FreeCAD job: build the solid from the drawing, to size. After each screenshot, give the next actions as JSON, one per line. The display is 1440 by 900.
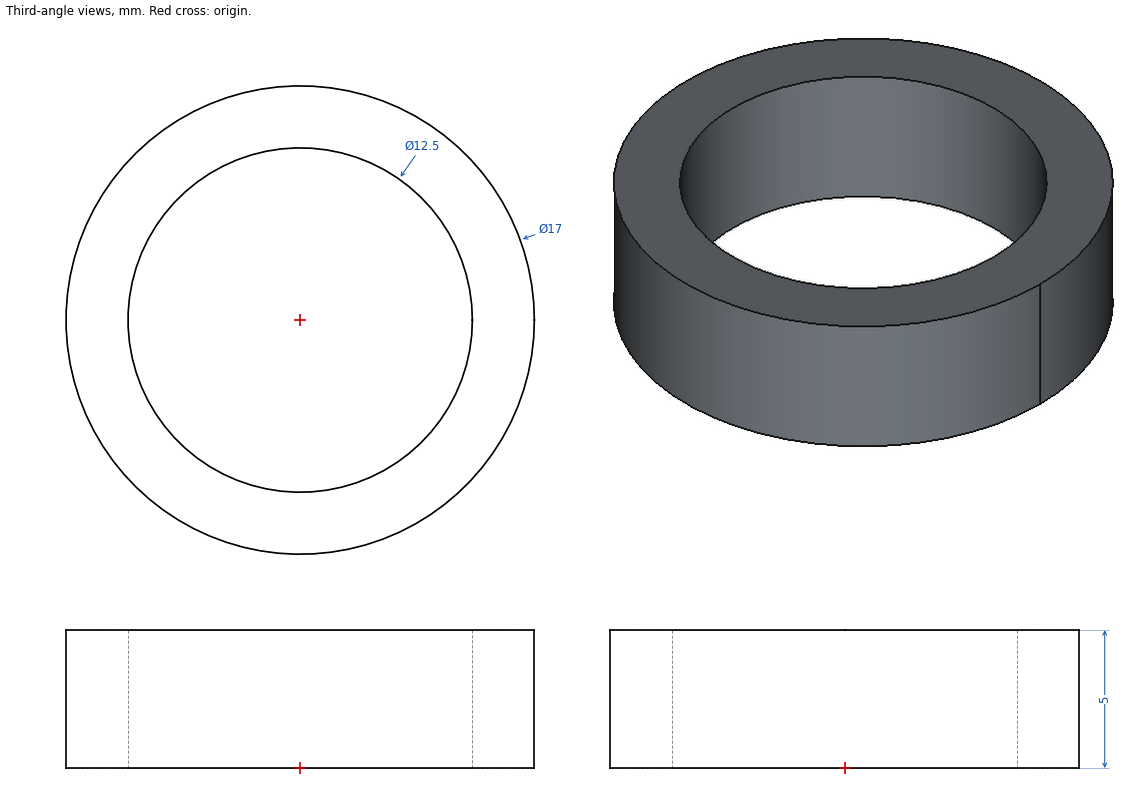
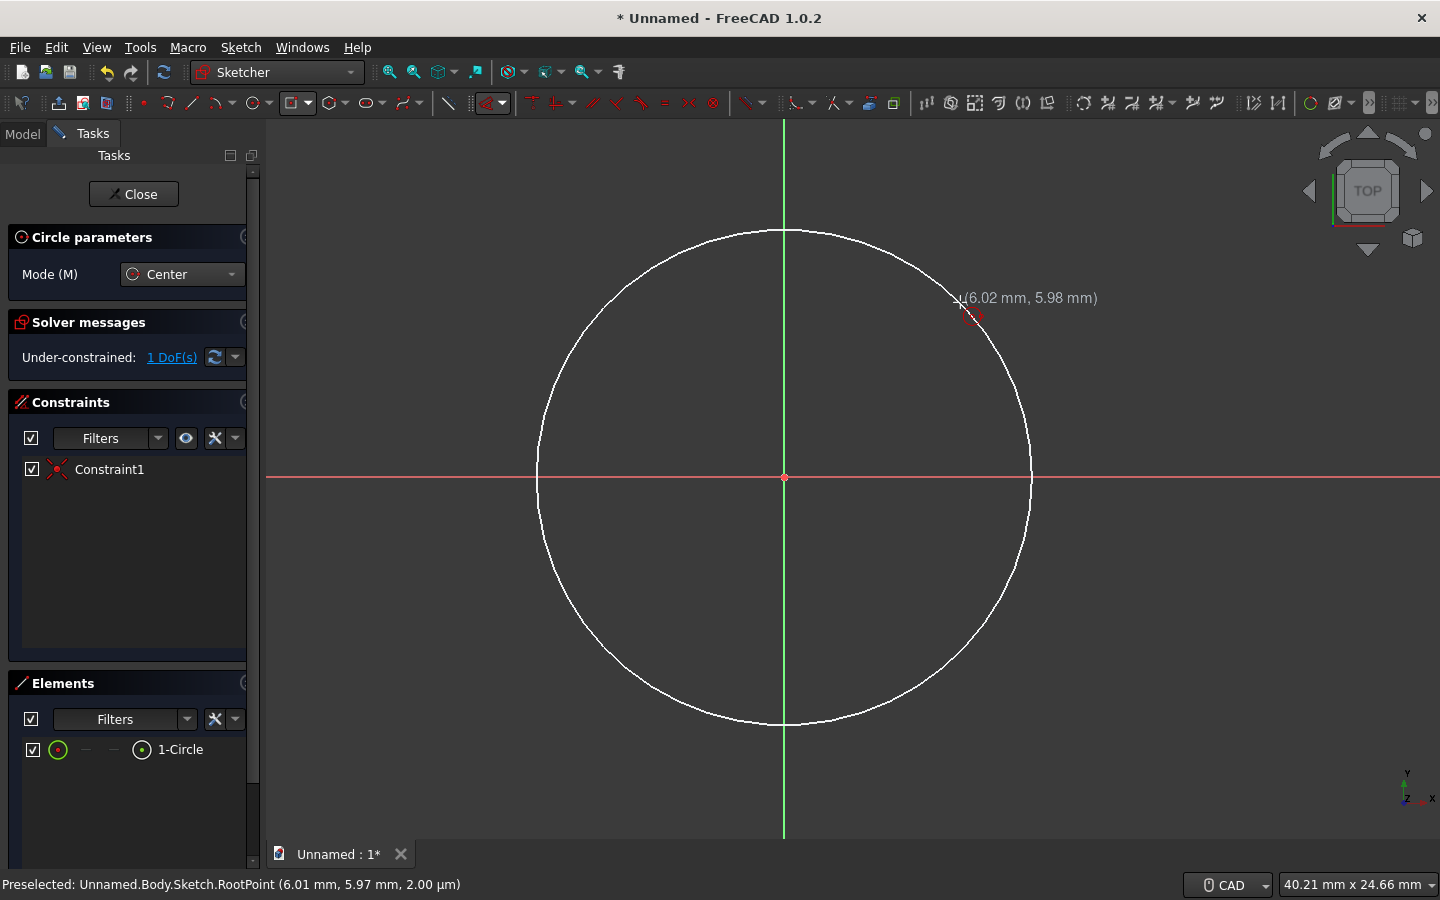
{"action": "left_click", "coordinate": [784, 477]}
{"action": "left_click", "coordinate": [913, 348]}
{"action": "key", "text": "Escape"}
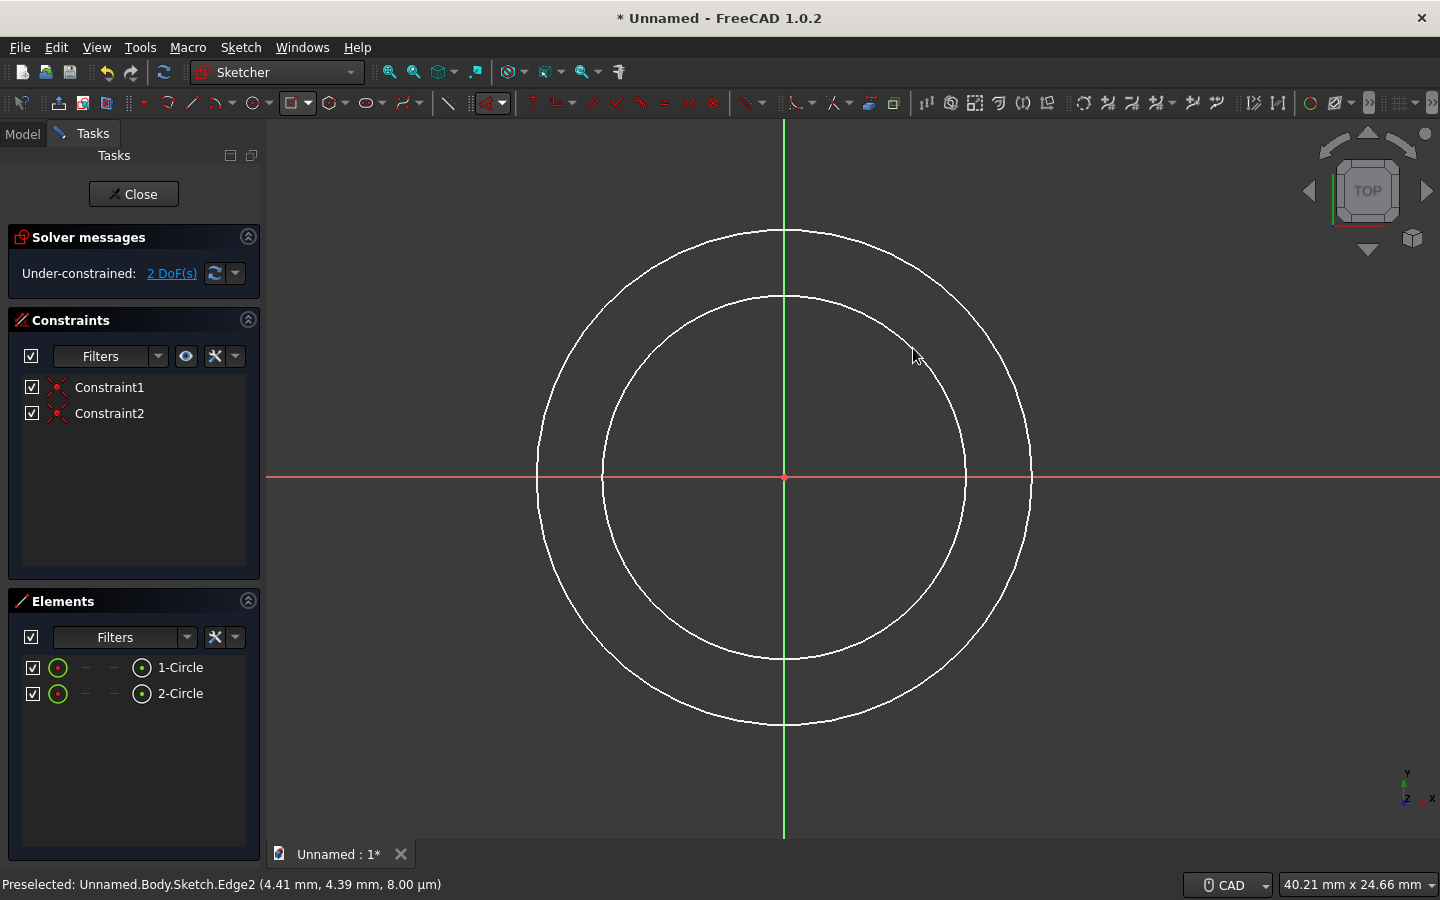
{"action": "key", "text": "d"}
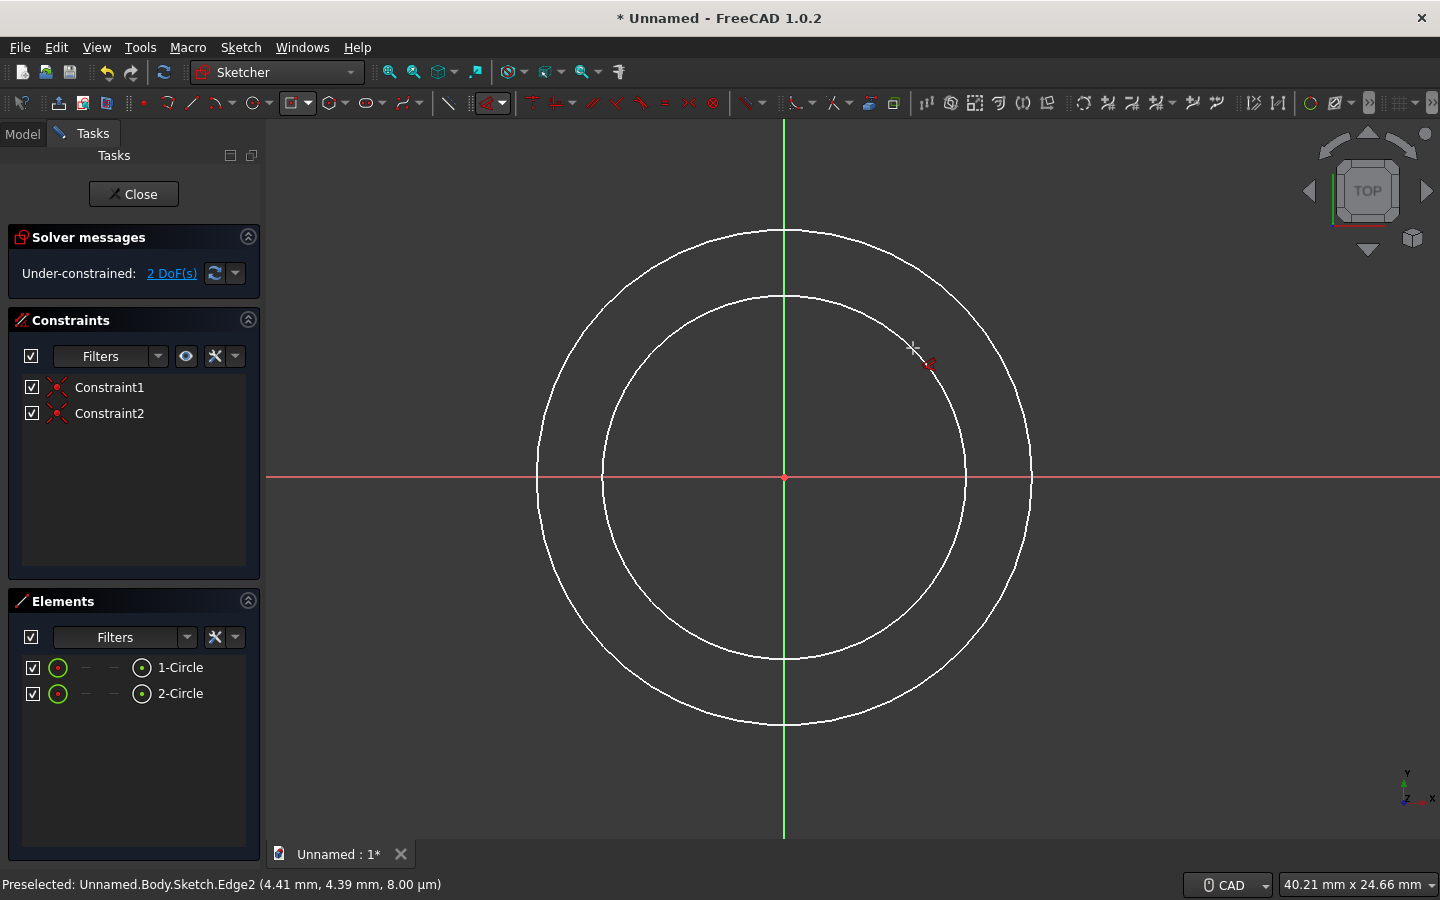
{"action": "left_click", "coordinate": [959, 302]}
{"action": "left_click", "coordinate": [982, 279]}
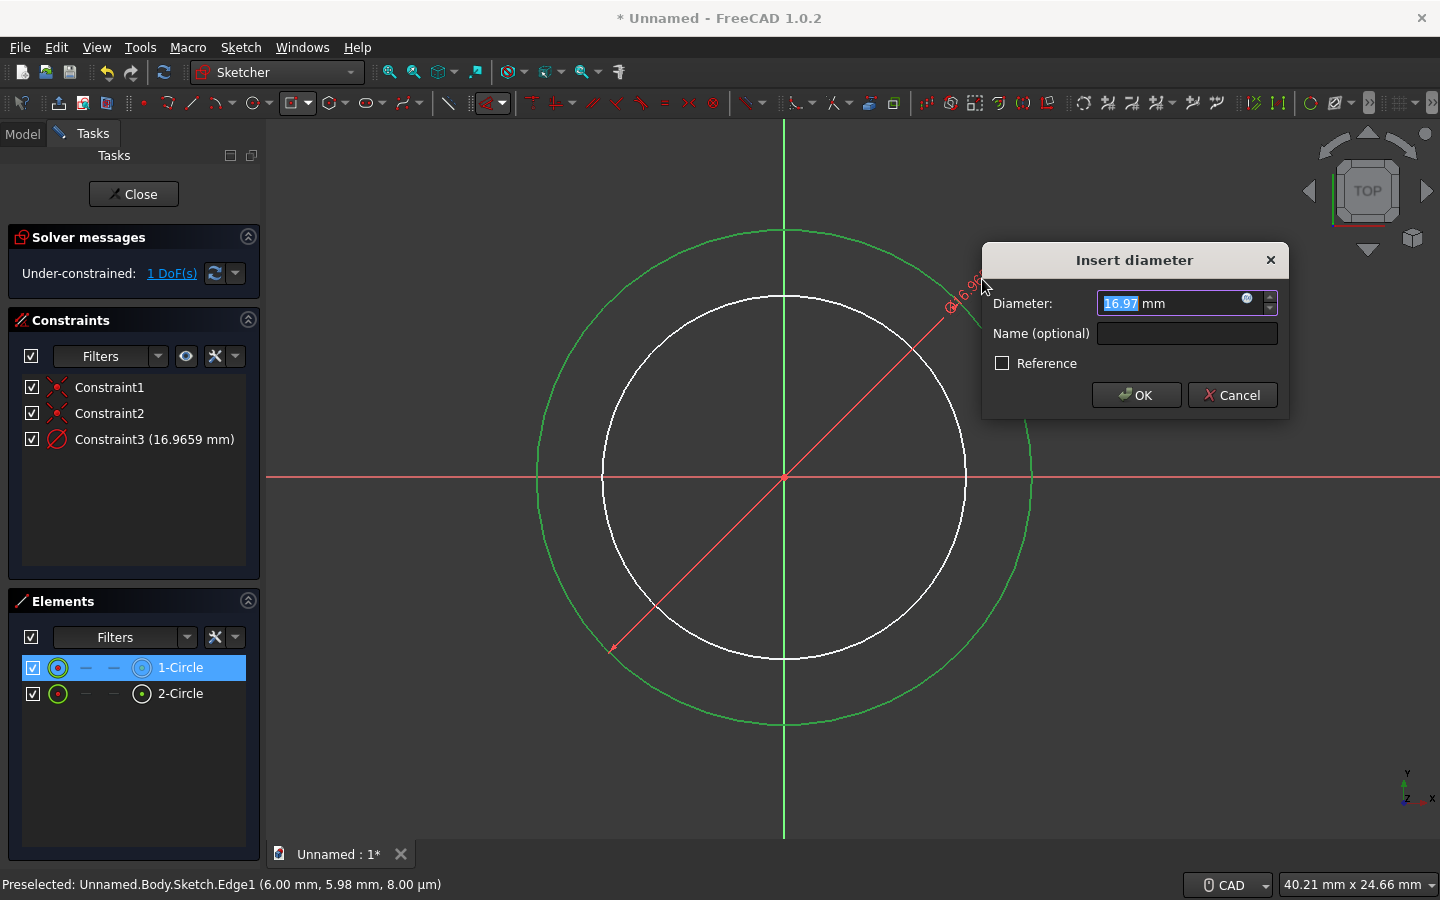
{"action": "type", "text": "17"}
{"action": "key", "text": "Return"}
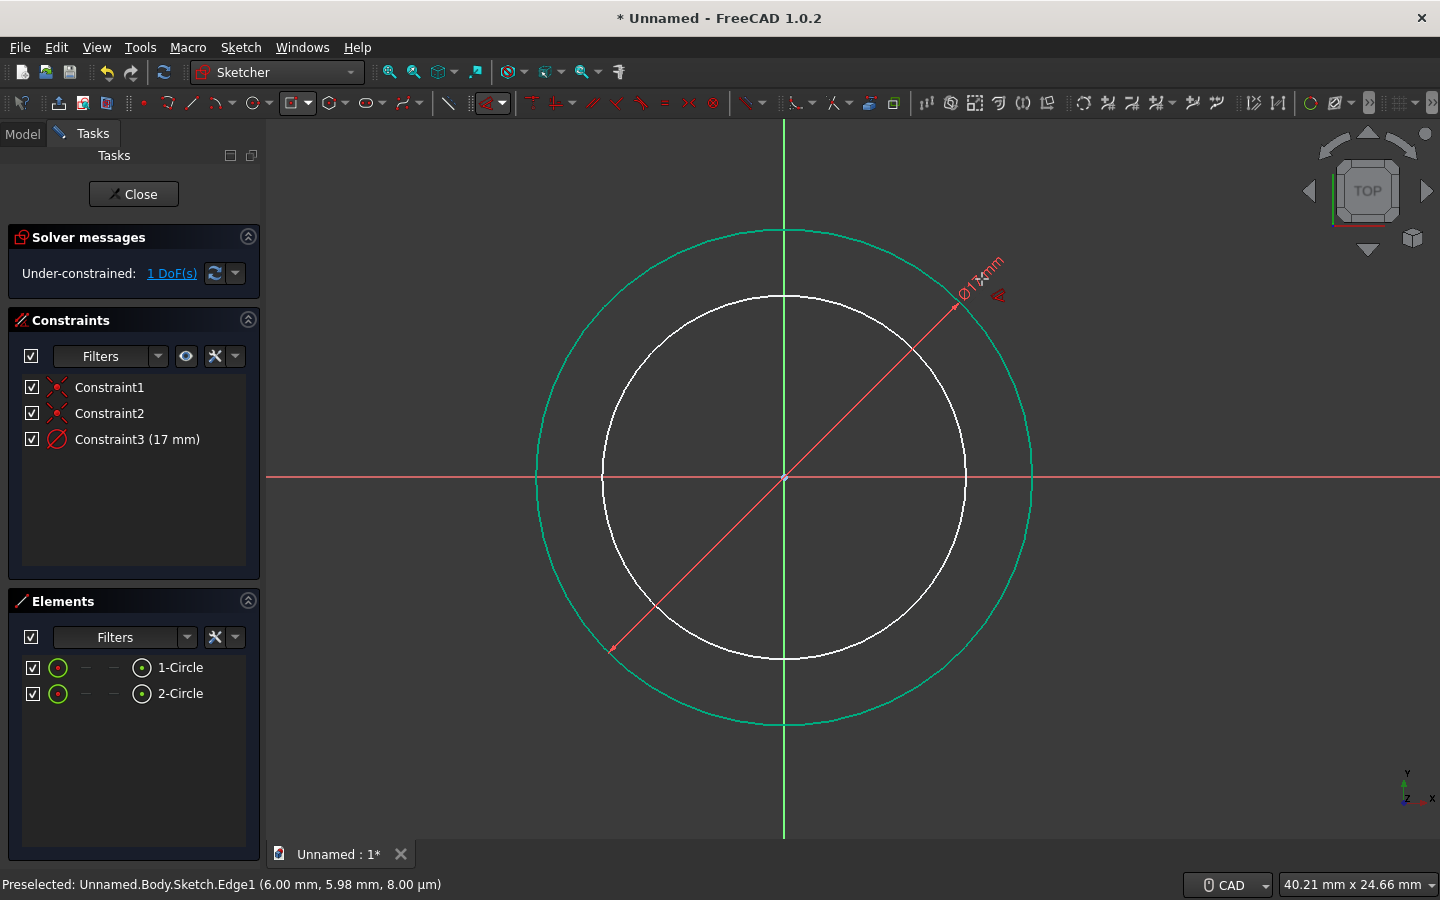
{"action": "left_click", "coordinate": [912, 348]}
{"action": "left_click", "coordinate": [934, 325]}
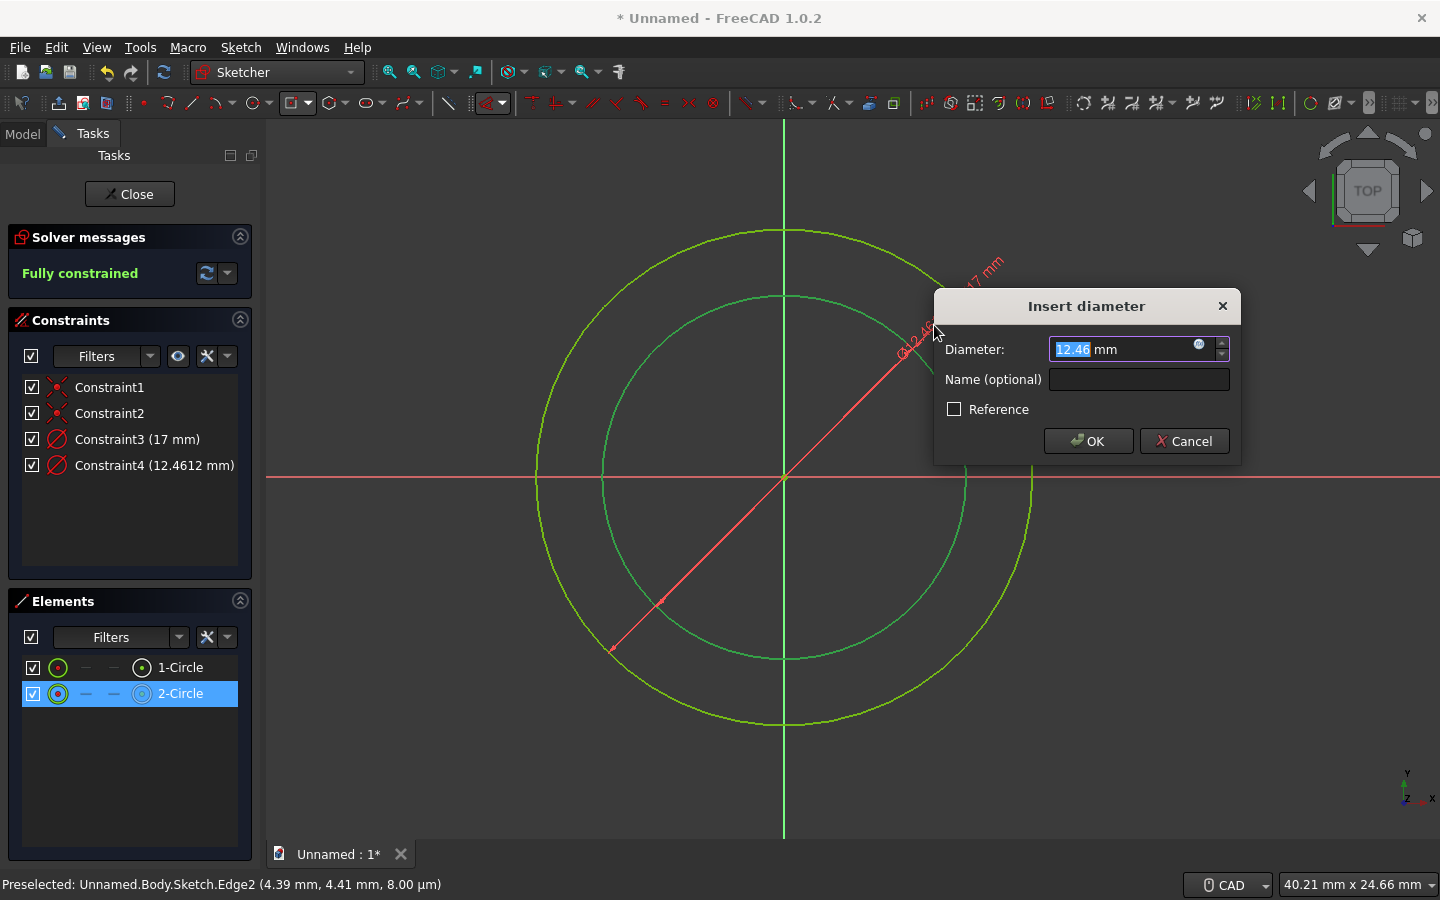
{"action": "type", "text": "12.5"}
{"action": "key", "text": "Return"}
{"action": "key", "text": "Escape"}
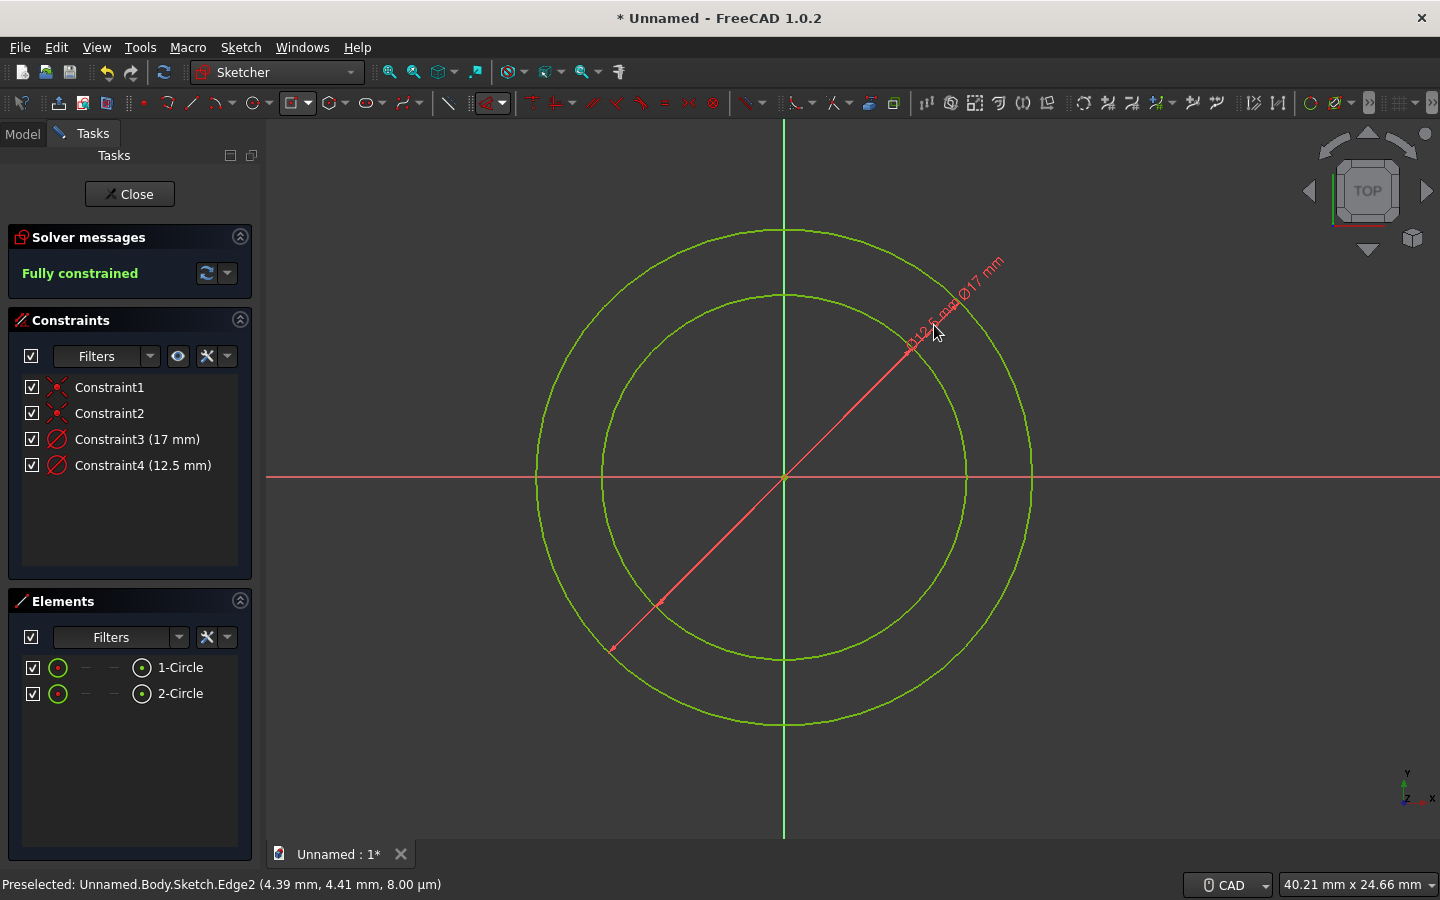
{"action": "left_click", "coordinate": [130, 194]}